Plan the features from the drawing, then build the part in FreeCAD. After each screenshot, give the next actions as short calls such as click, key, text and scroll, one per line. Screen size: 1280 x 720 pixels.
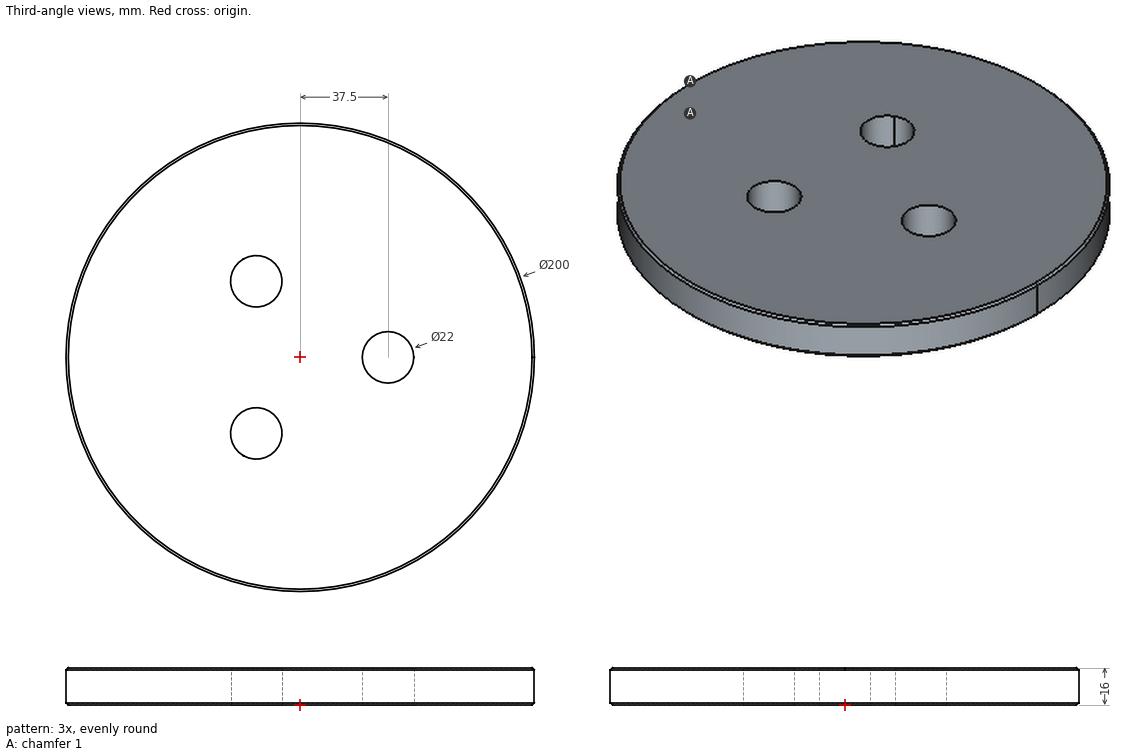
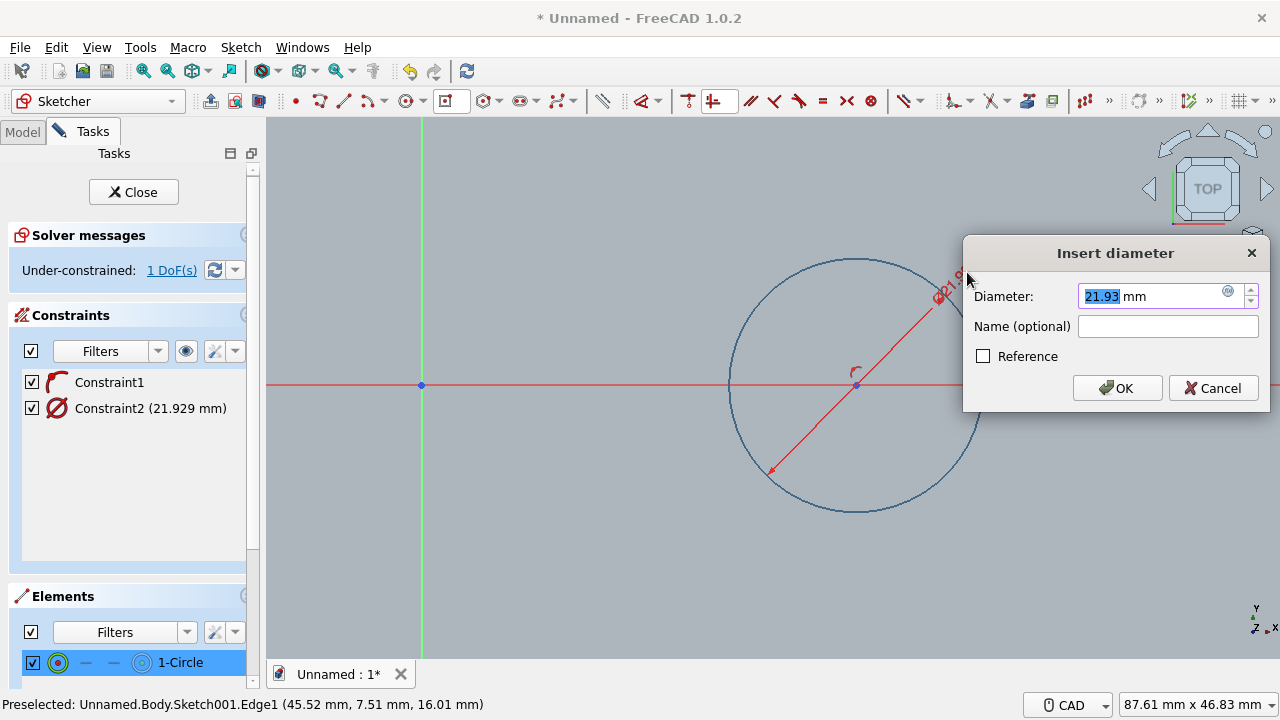
text(22)
key(Return)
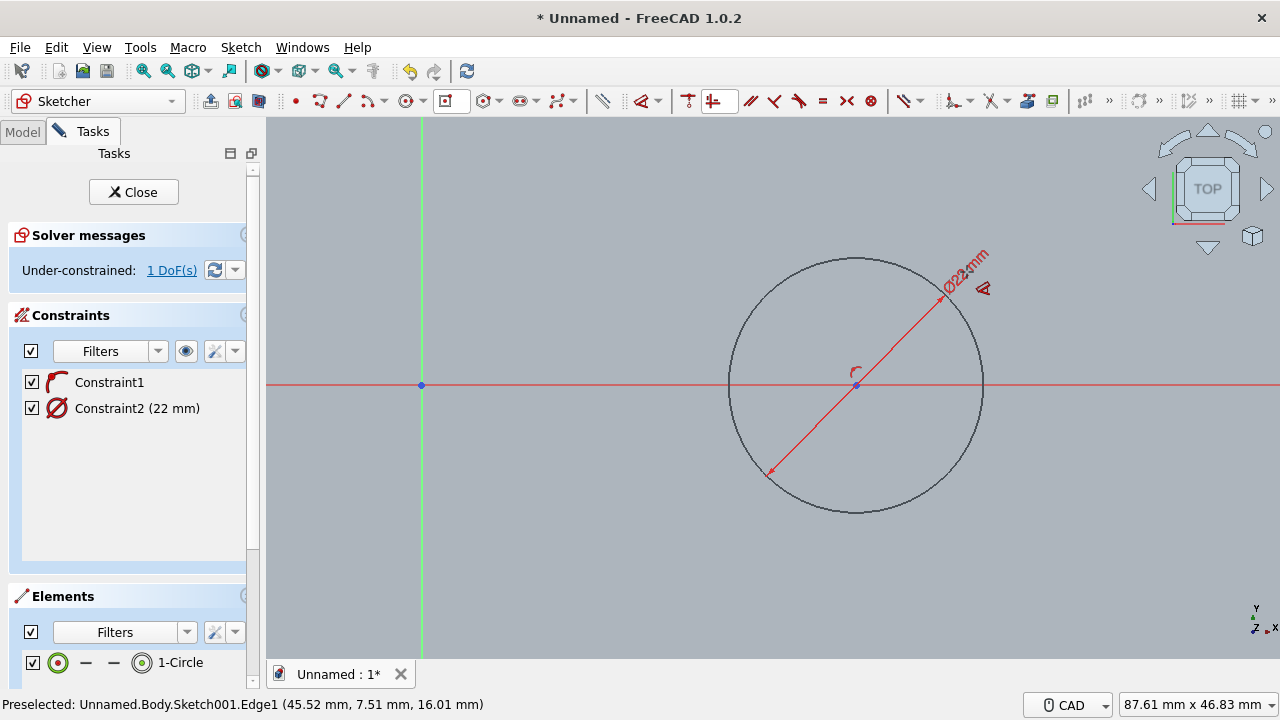
click(856, 385)
click(639, 419)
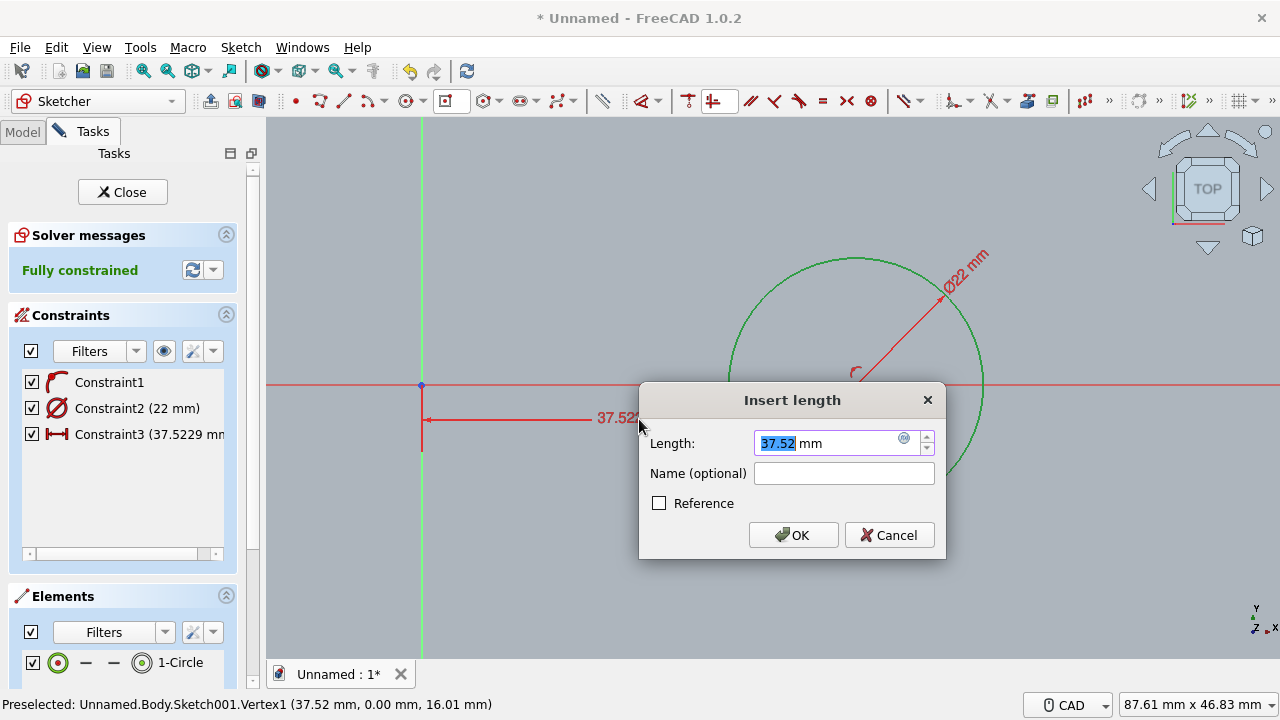
text(37.5)
key(Return)
key(Escape)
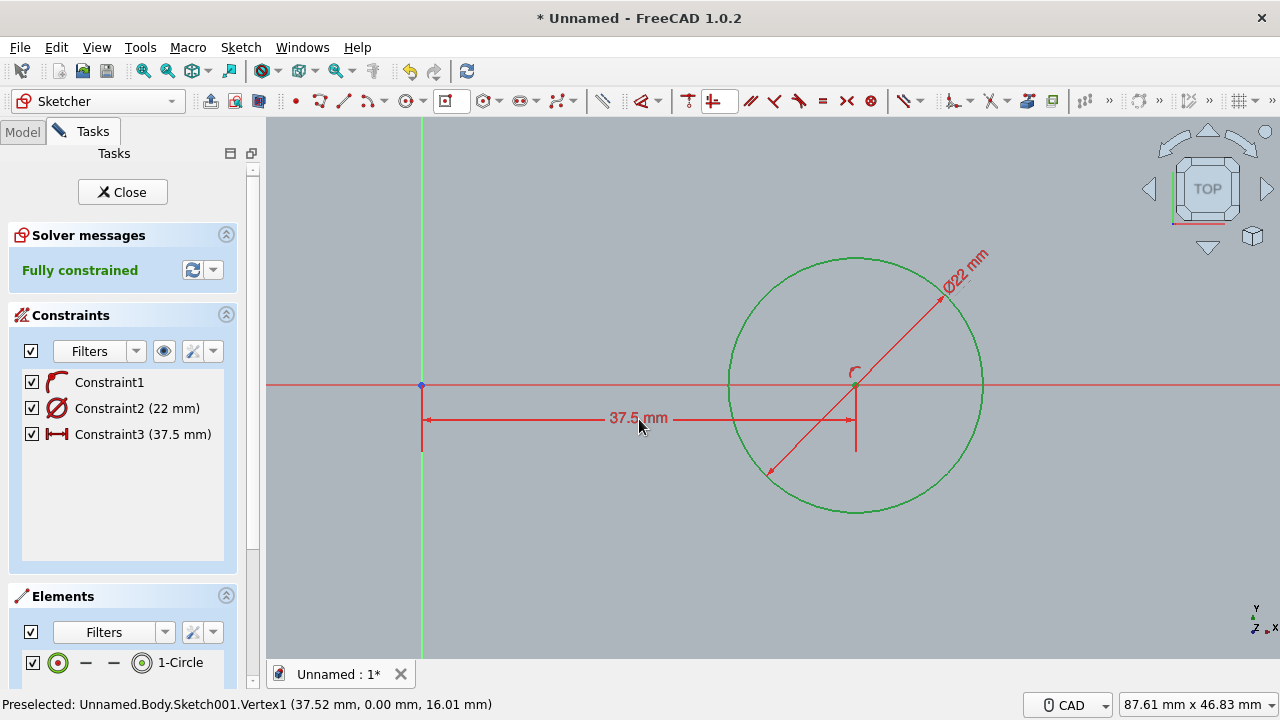
click(123, 192)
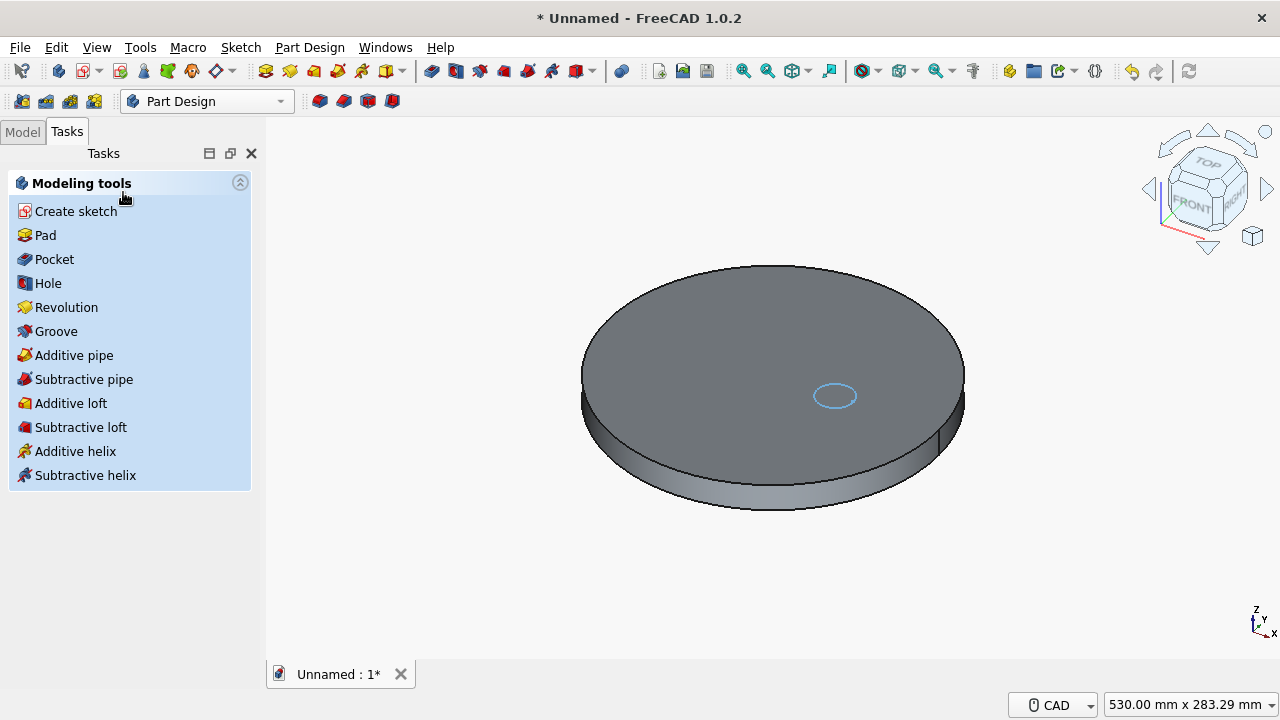
click(432, 72)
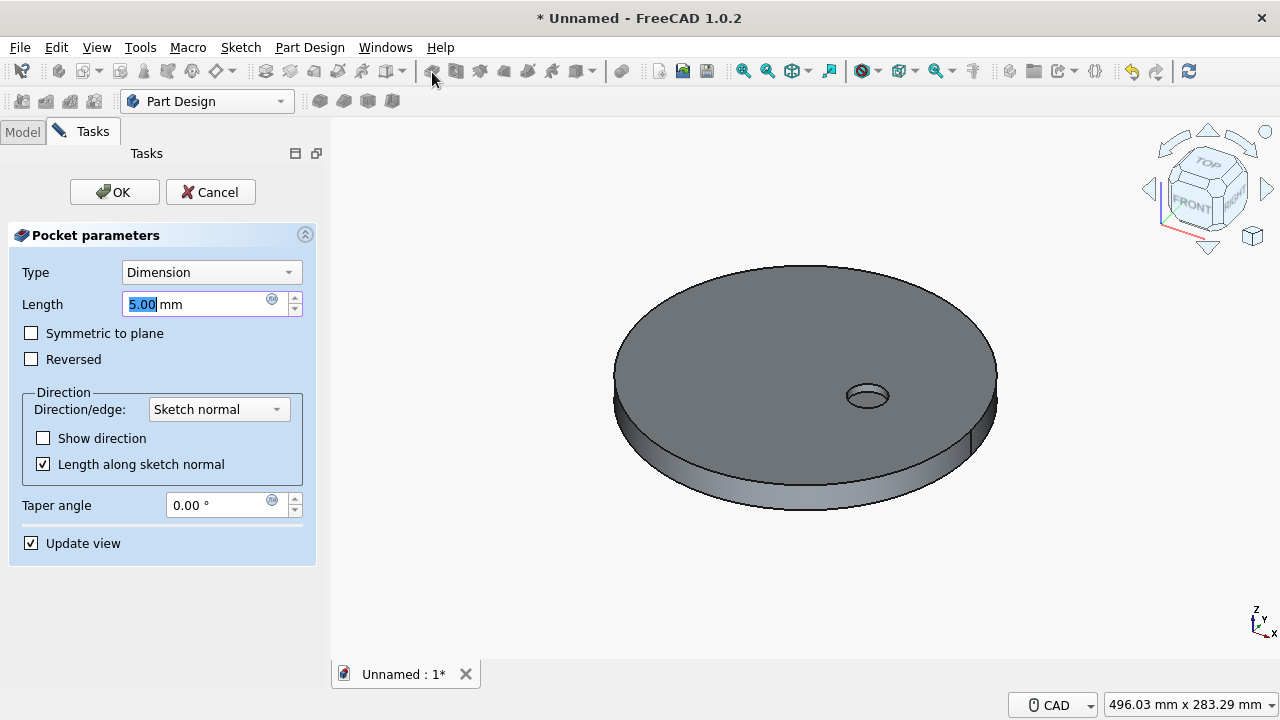
click(212, 272)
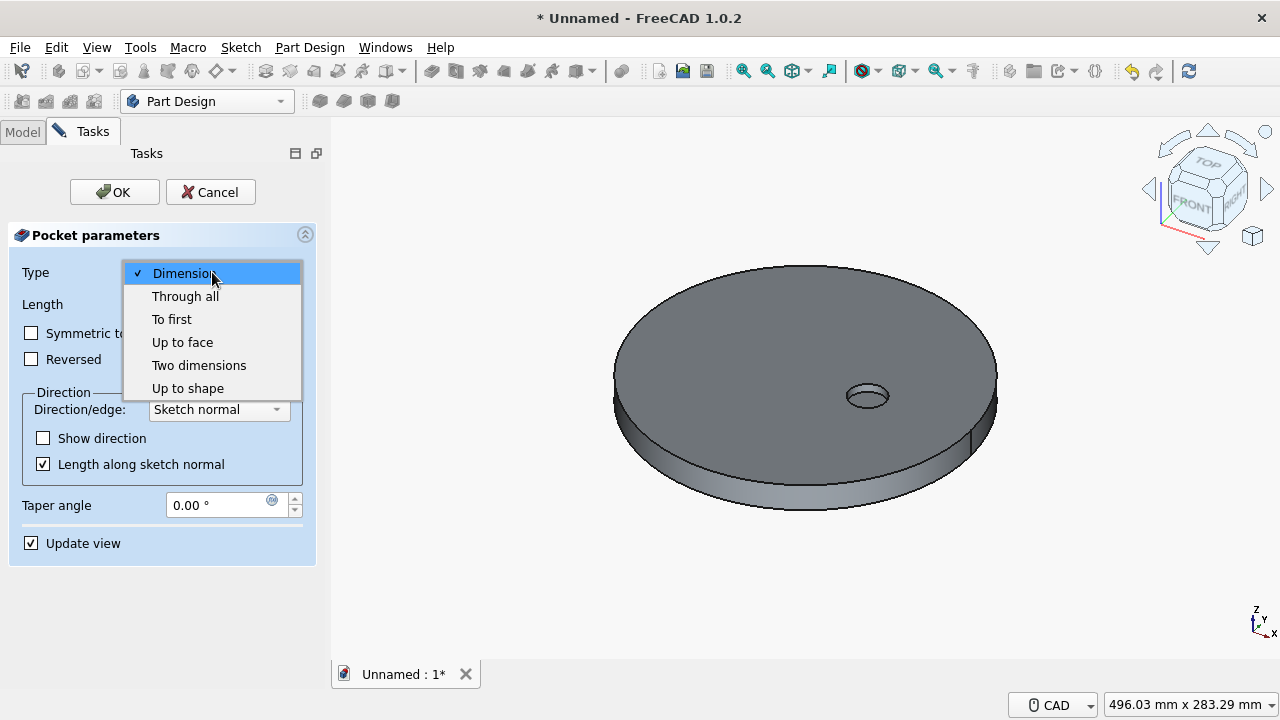
click(212, 296)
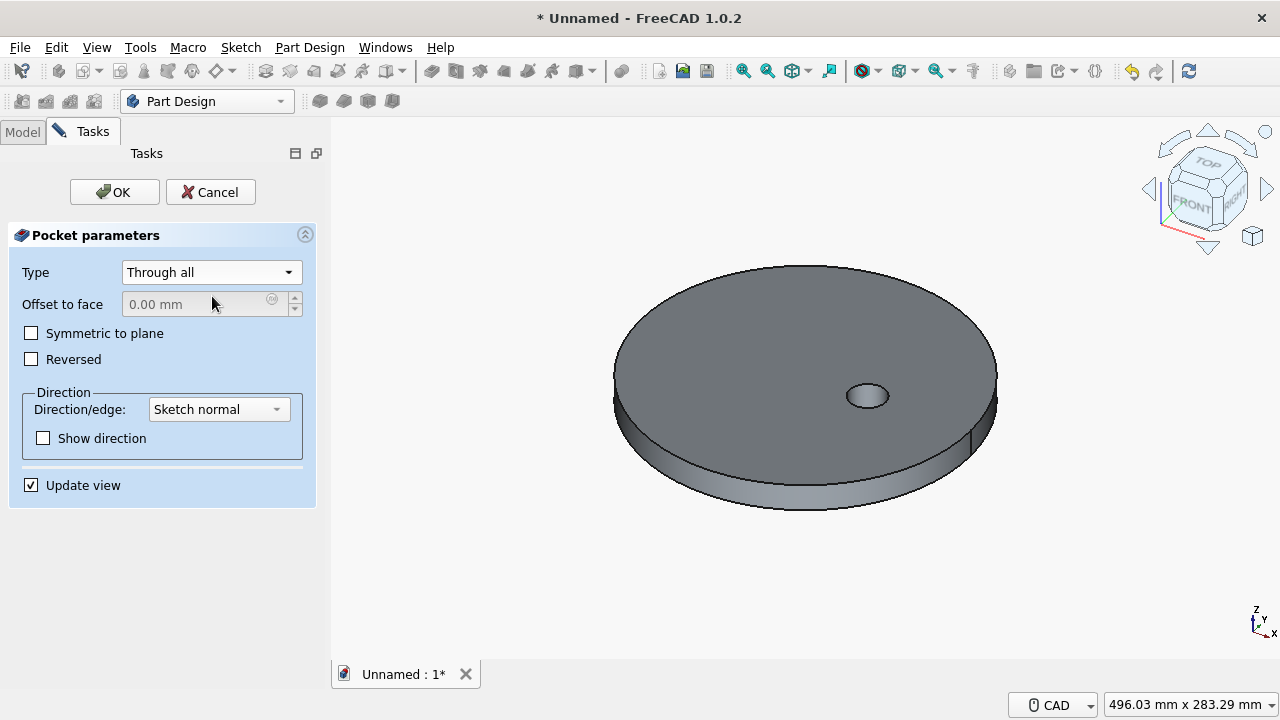
click(115, 192)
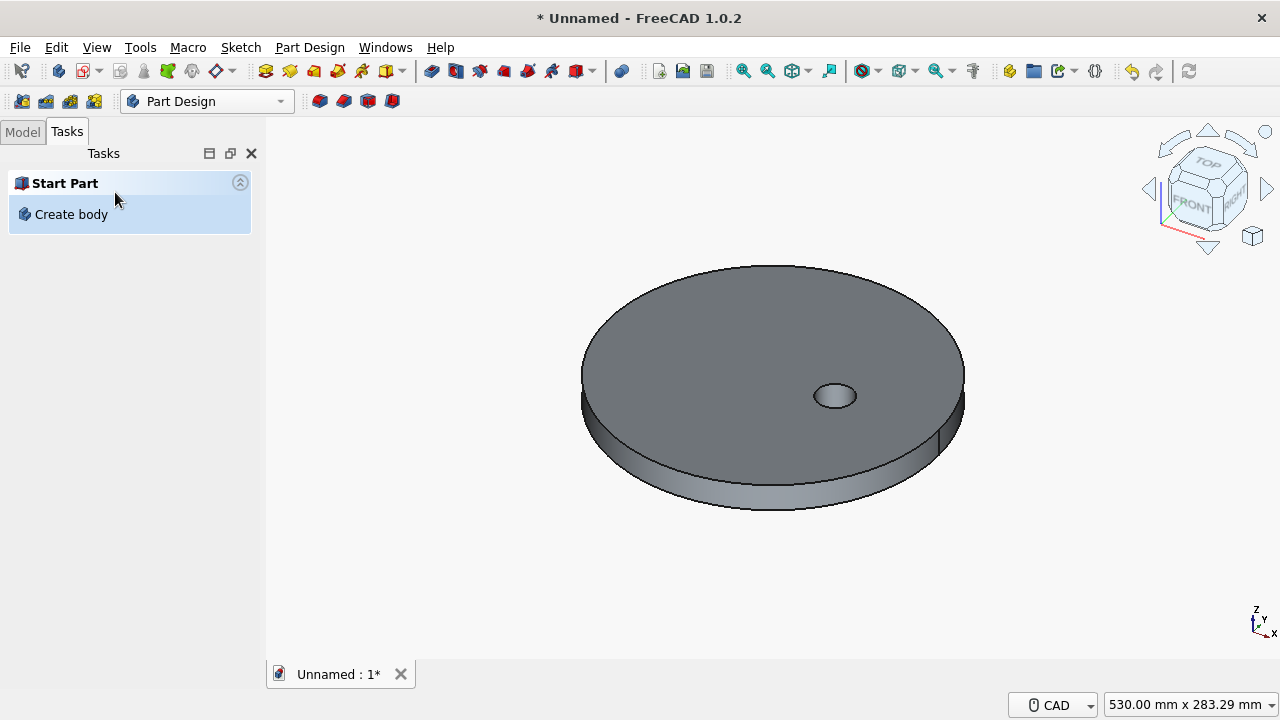
click(23, 131)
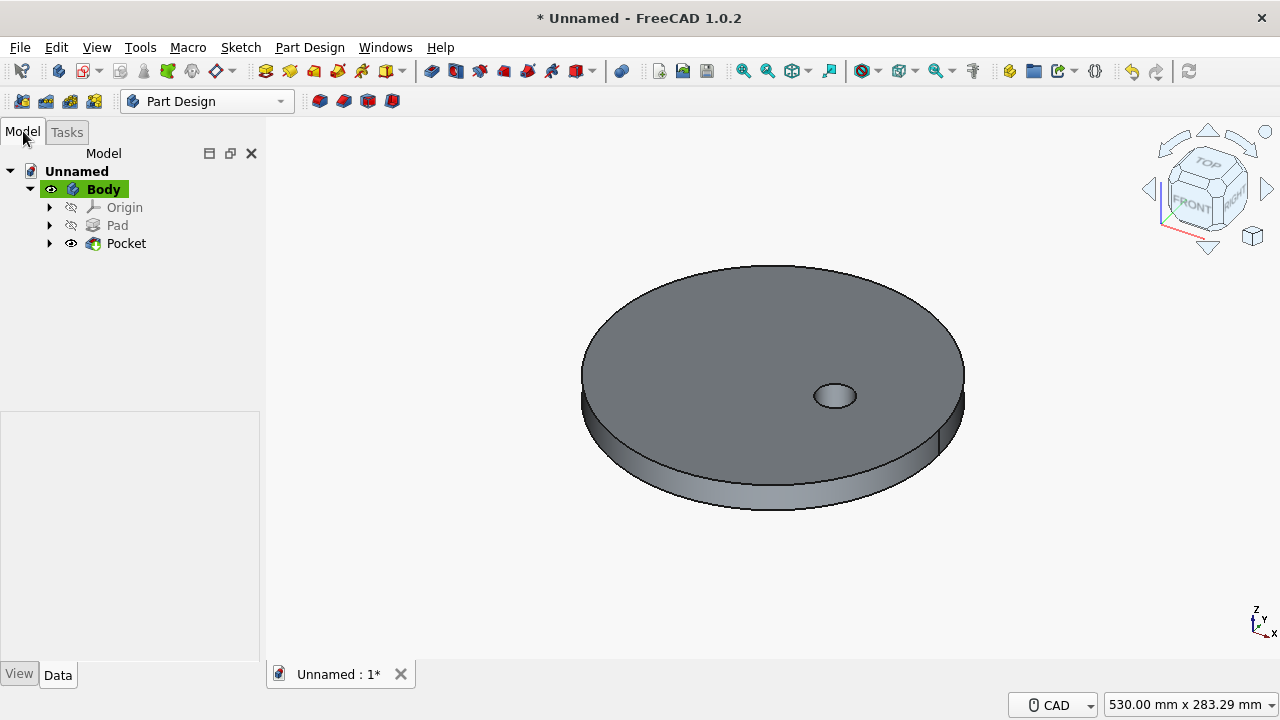
click(116, 243)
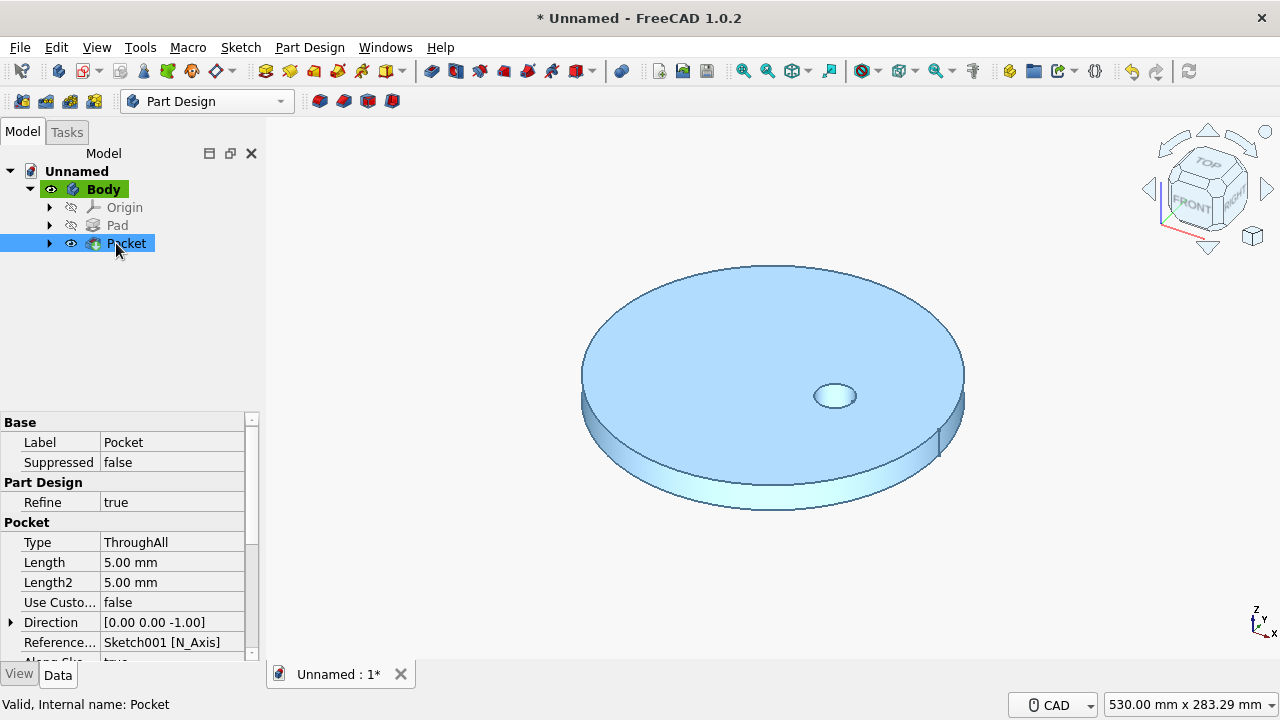
click(70, 102)